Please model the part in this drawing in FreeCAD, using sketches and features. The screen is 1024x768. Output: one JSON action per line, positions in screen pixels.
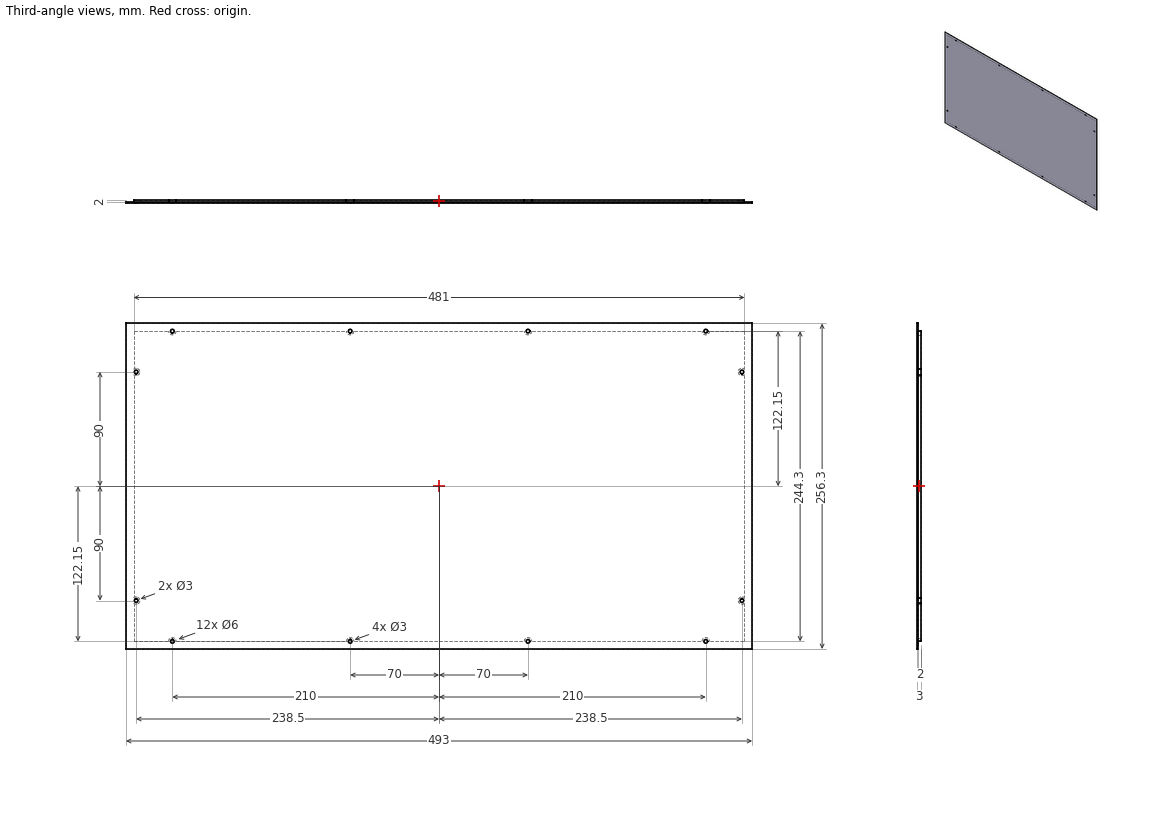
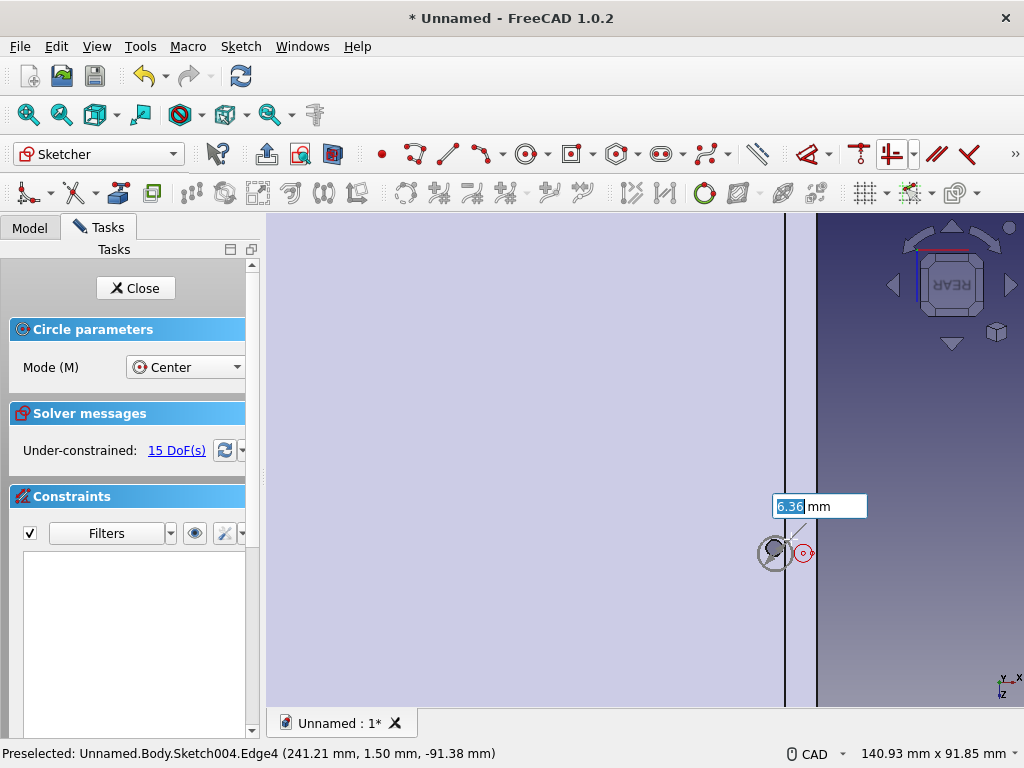
{"action": "left_click", "coordinate": [786, 537]}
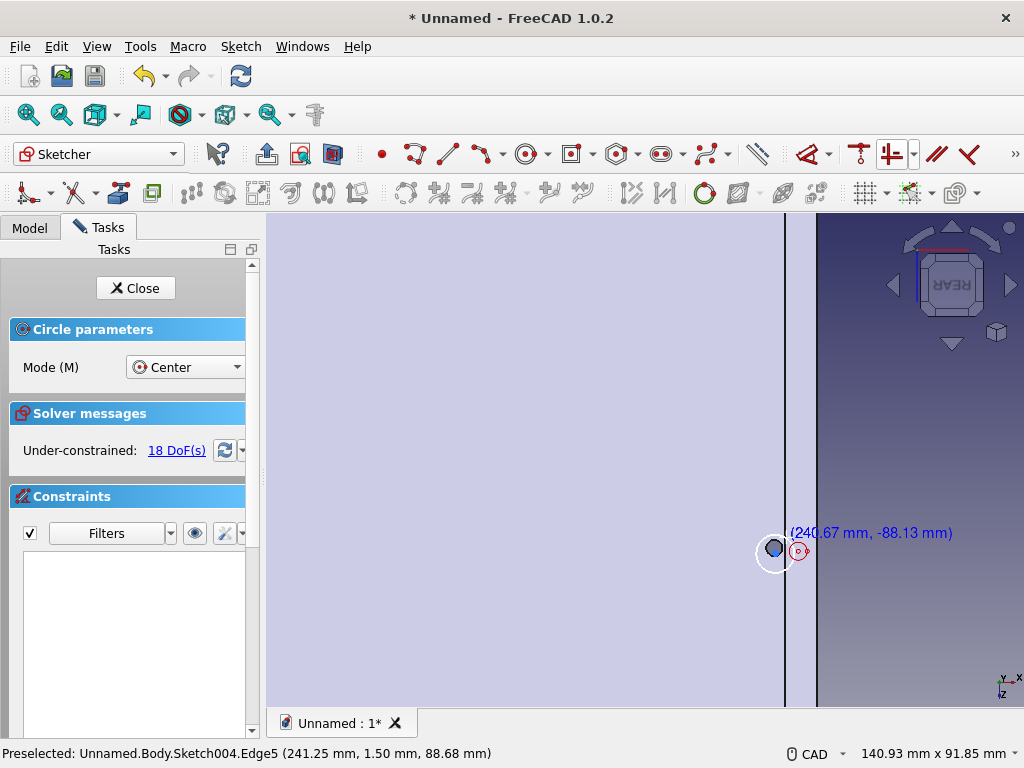
{"action": "scroll", "coordinate": [791, 538], "scroll_direction": "down", "scroll_amount": 9}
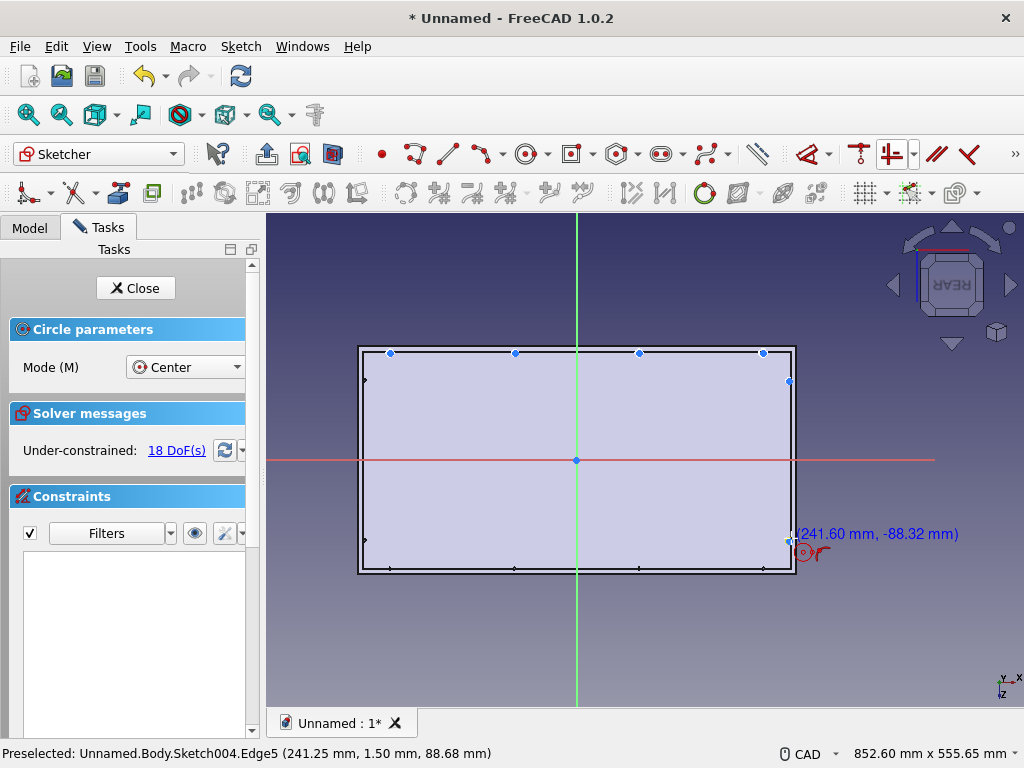
{"action": "scroll", "coordinate": [763, 569], "scroll_direction": "up", "scroll_amount": 11}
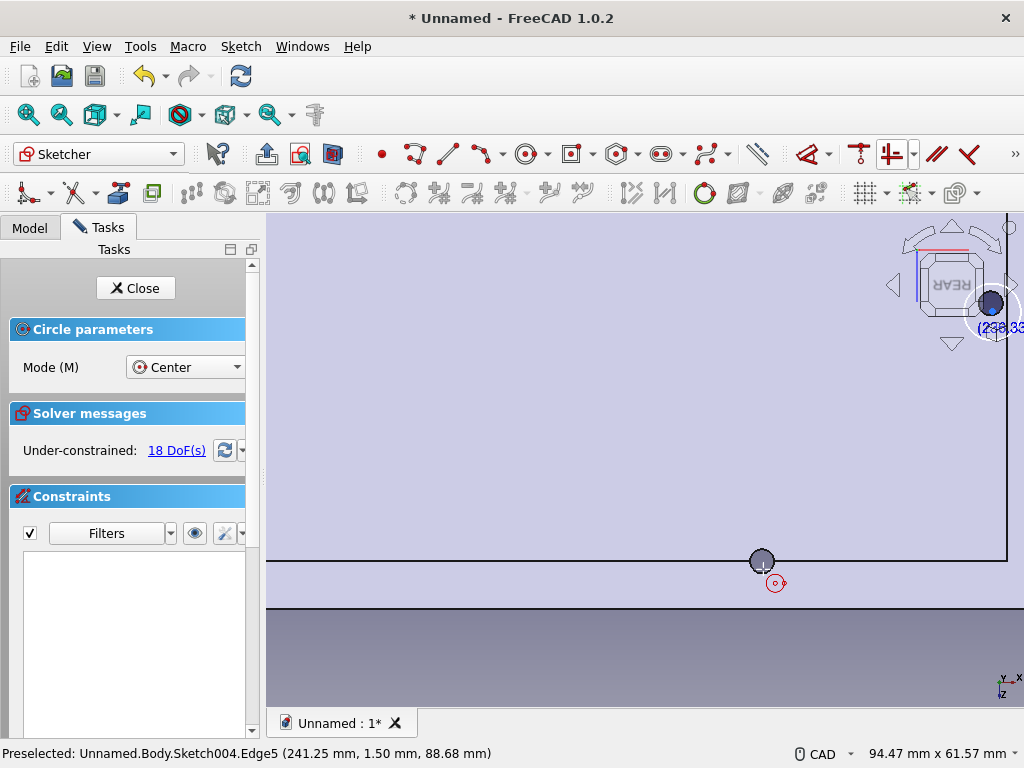
{"action": "scroll", "coordinate": [763, 570], "scroll_direction": "down", "scroll_amount": 11}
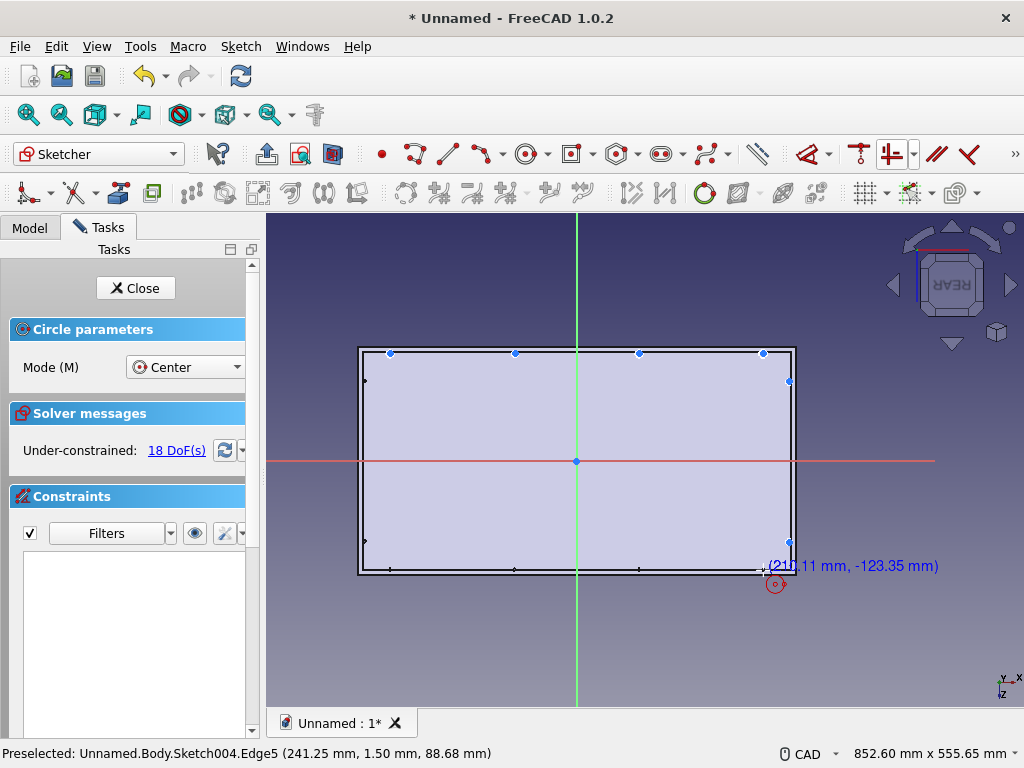
{"action": "left_click", "coordinate": [763, 570]}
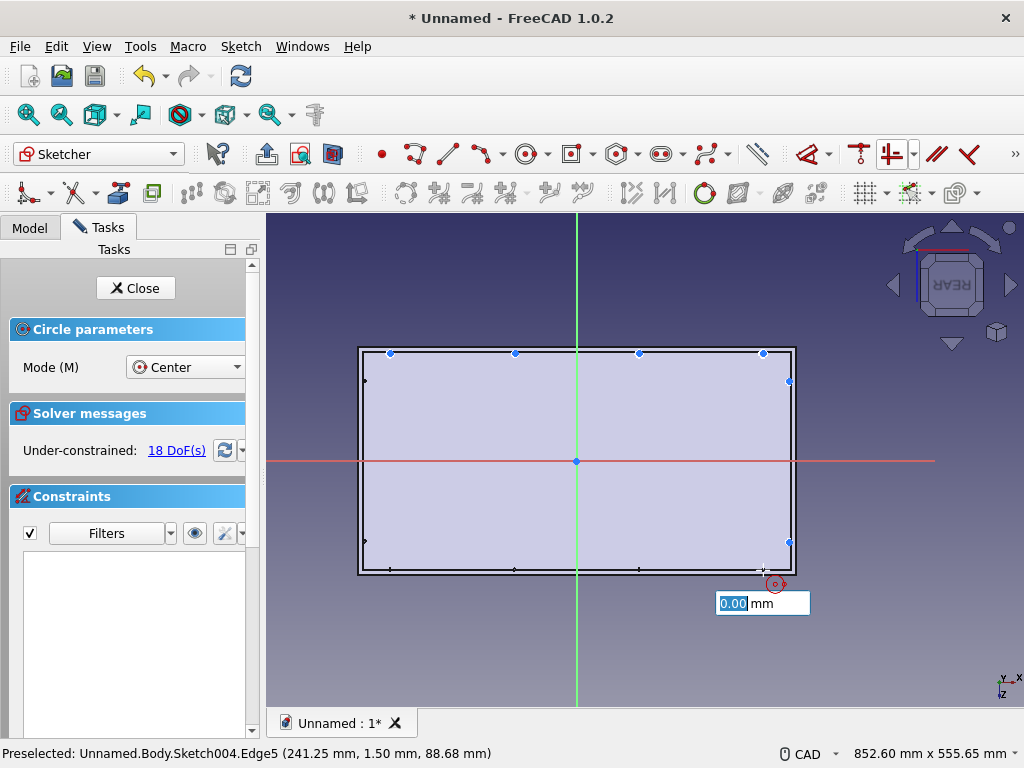
{"action": "scroll", "coordinate": [765, 568], "scroll_direction": "up", "scroll_amount": 9}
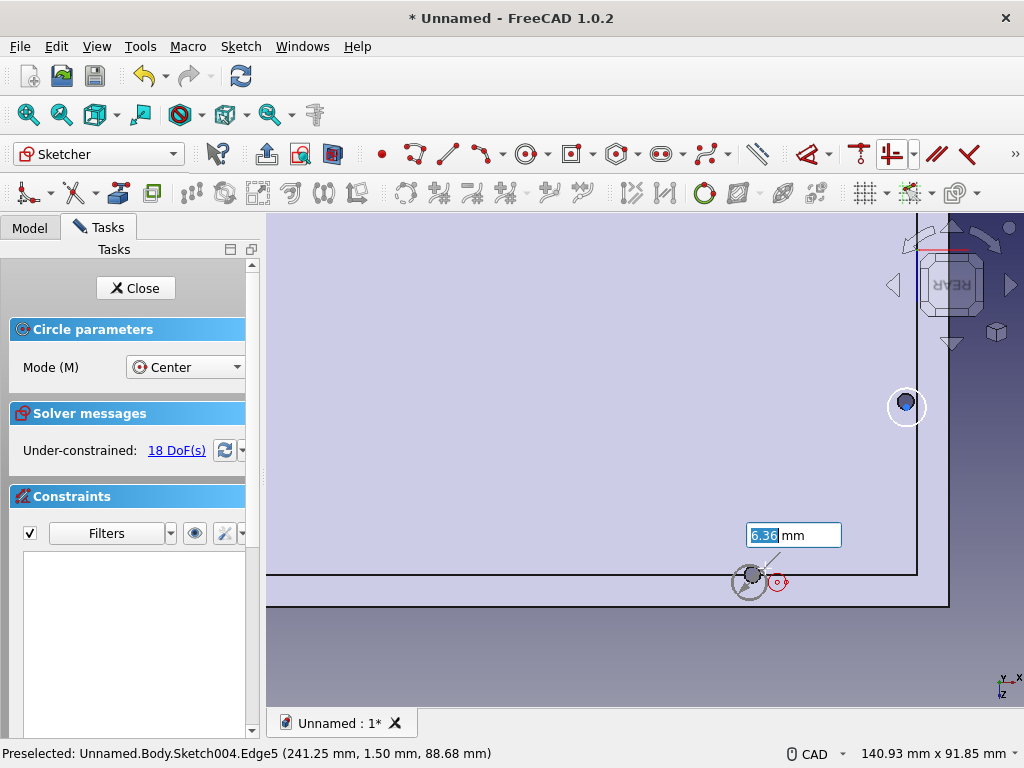
{"action": "left_click", "coordinate": [764, 563]}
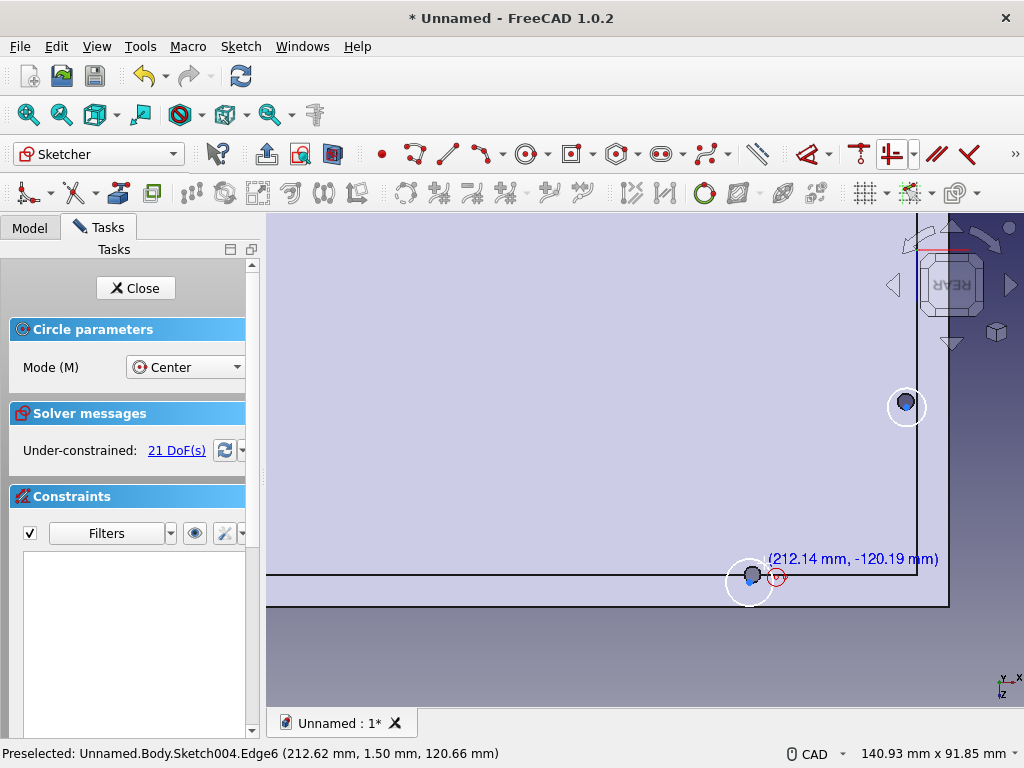
{"action": "scroll", "coordinate": [765, 567], "scroll_direction": "down", "scroll_amount": 9}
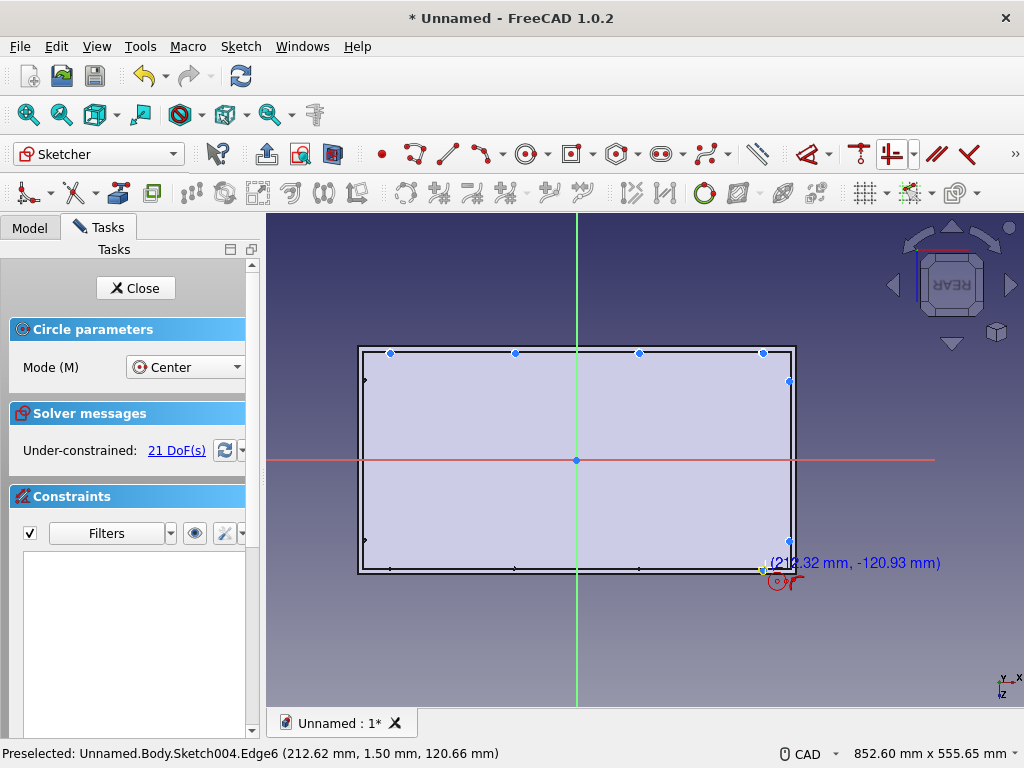
{"action": "scroll", "coordinate": [639, 569], "scroll_direction": "up", "scroll_amount": 11}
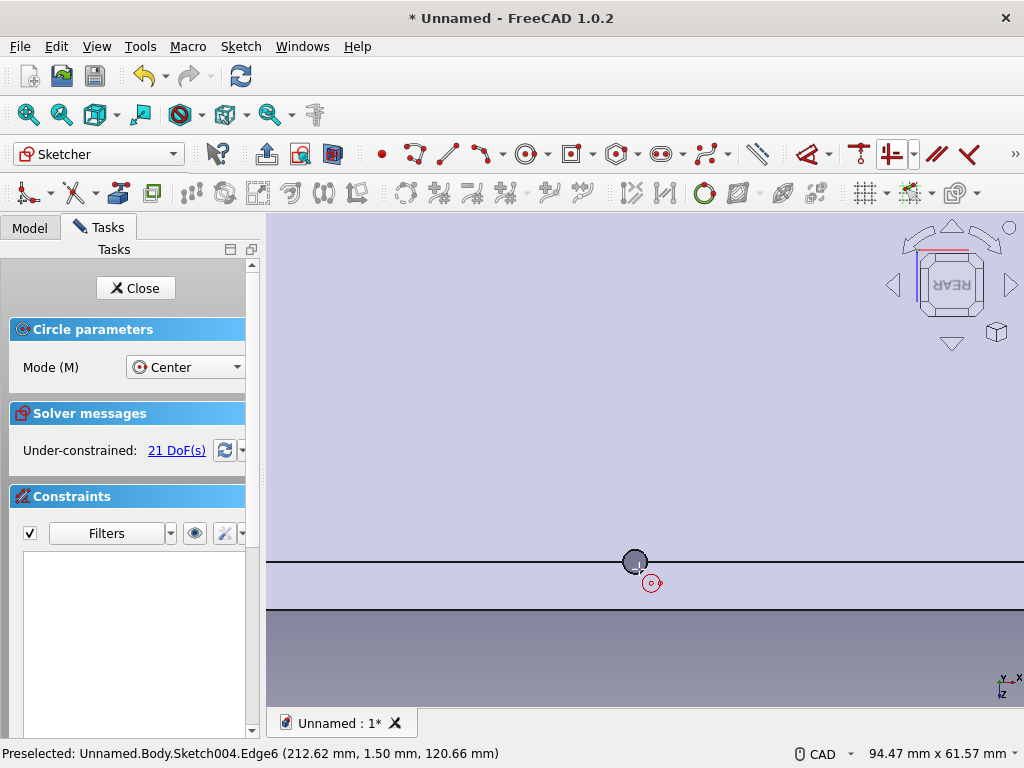
{"action": "scroll", "coordinate": [639, 569], "scroll_direction": "down", "scroll_amount": 11}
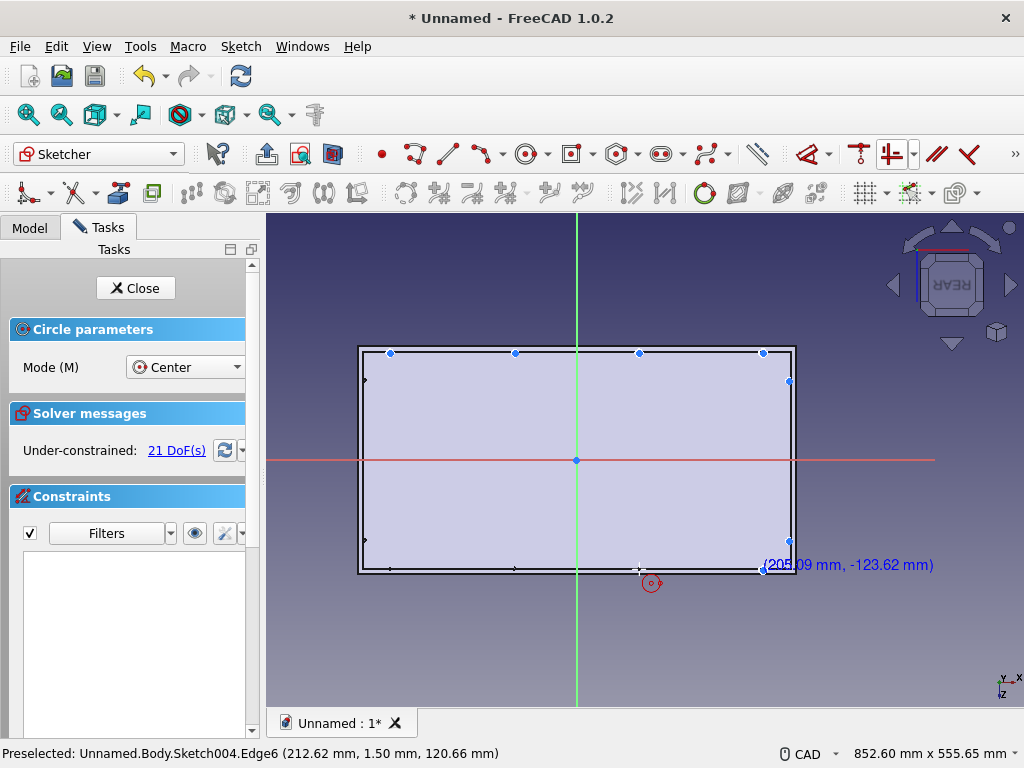
{"action": "left_click", "coordinate": [639, 569]}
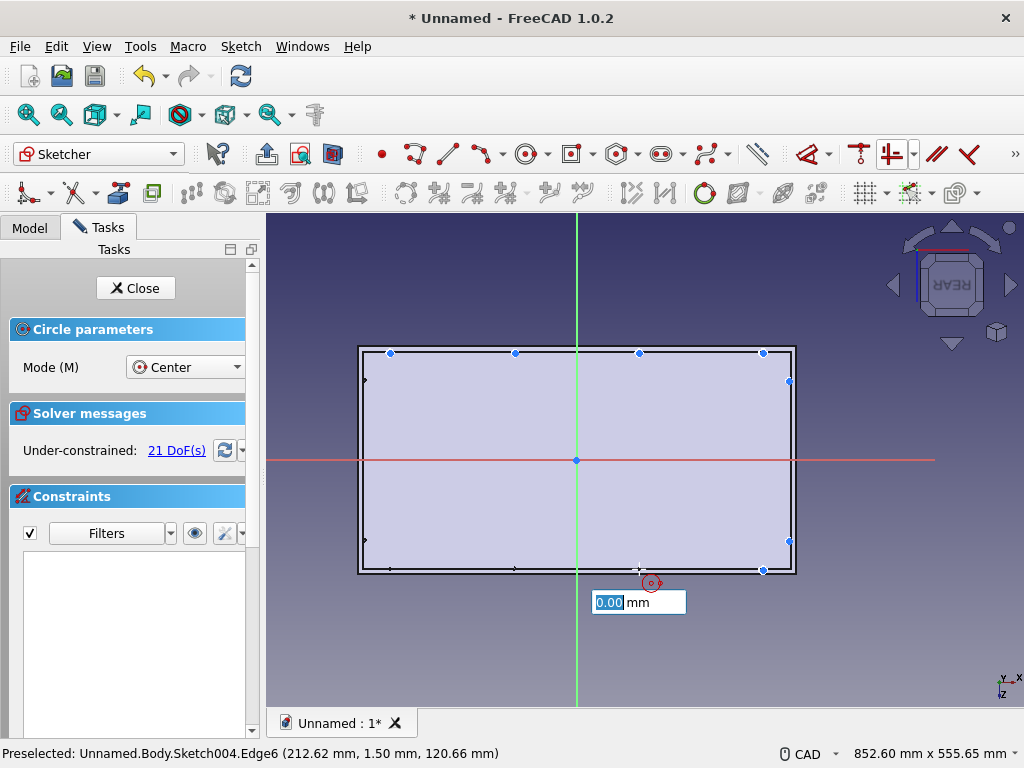
{"action": "scroll", "coordinate": [641, 567], "scroll_direction": "up", "scroll_amount": 9}